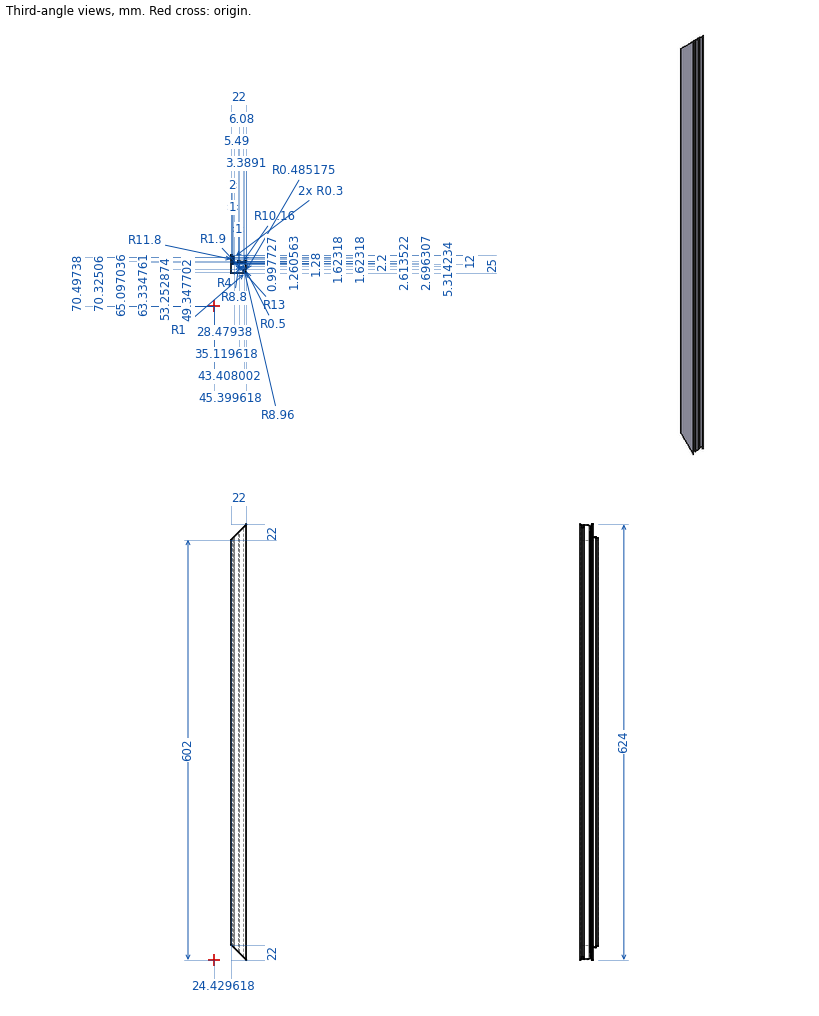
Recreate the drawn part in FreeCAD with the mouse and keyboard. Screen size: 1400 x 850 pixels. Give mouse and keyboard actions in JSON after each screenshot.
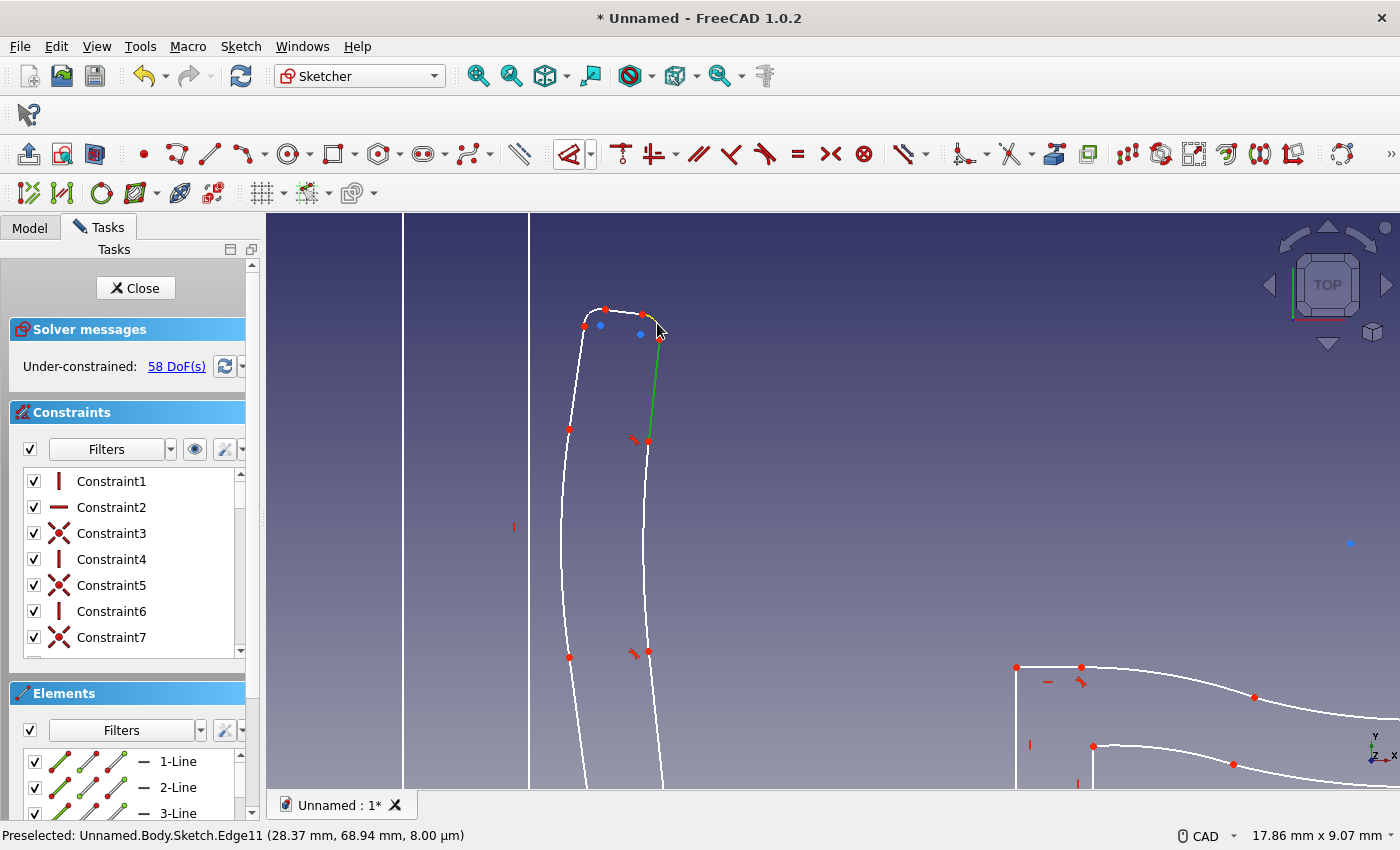
{"action": "left_click", "coordinate": [657, 323]}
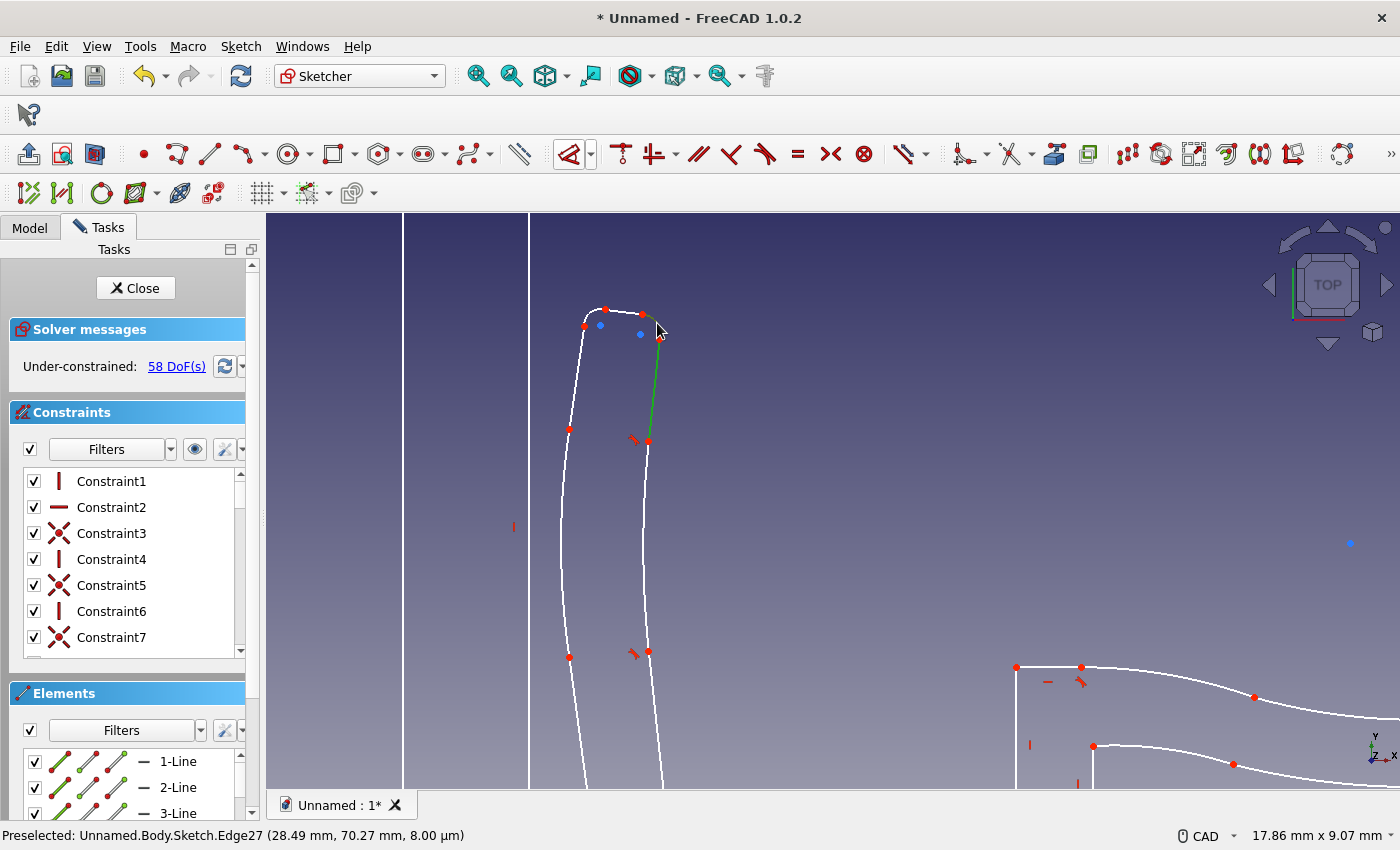
{"action": "key", "text": "t"}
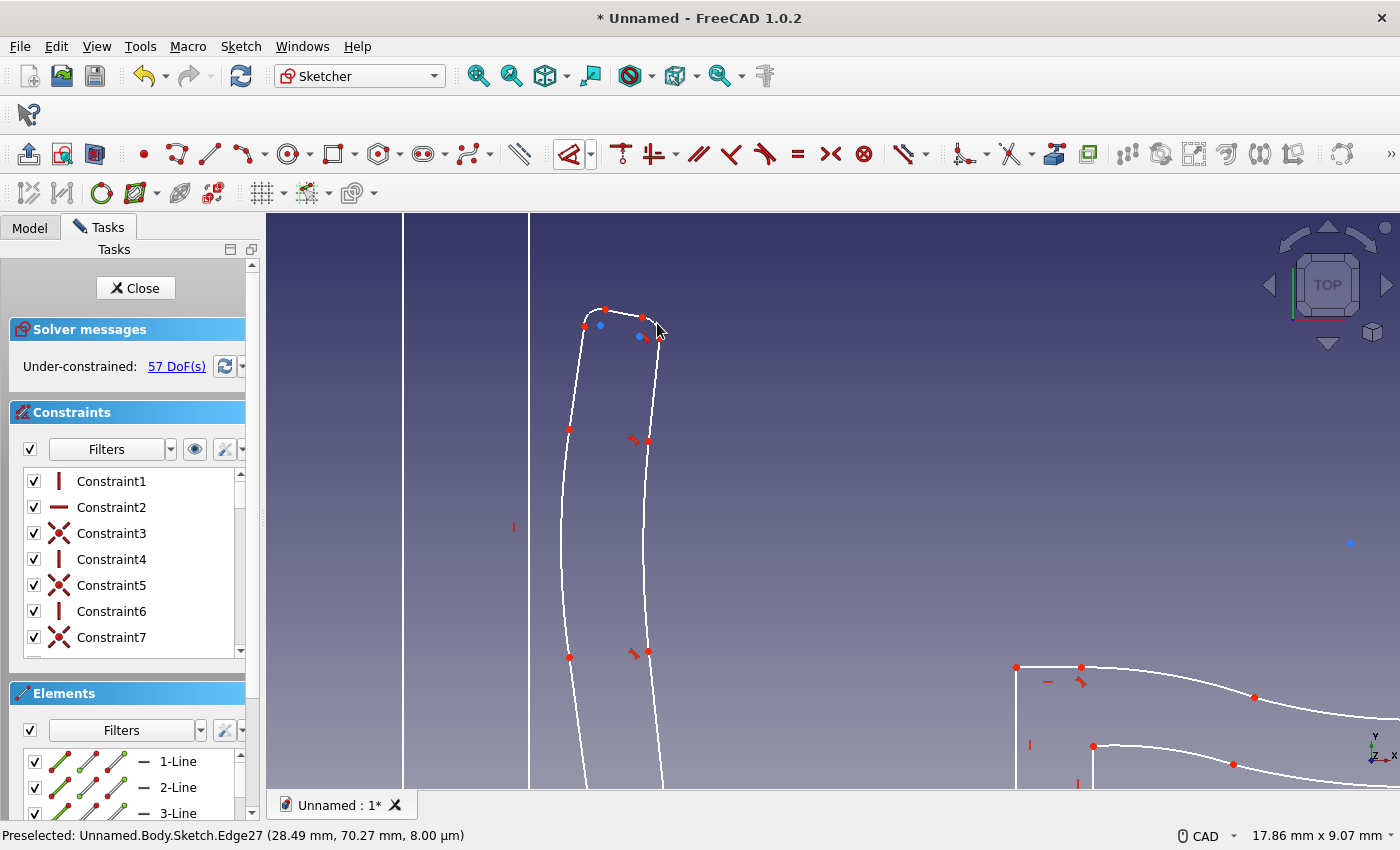
{"action": "left_click", "coordinate": [631, 315]}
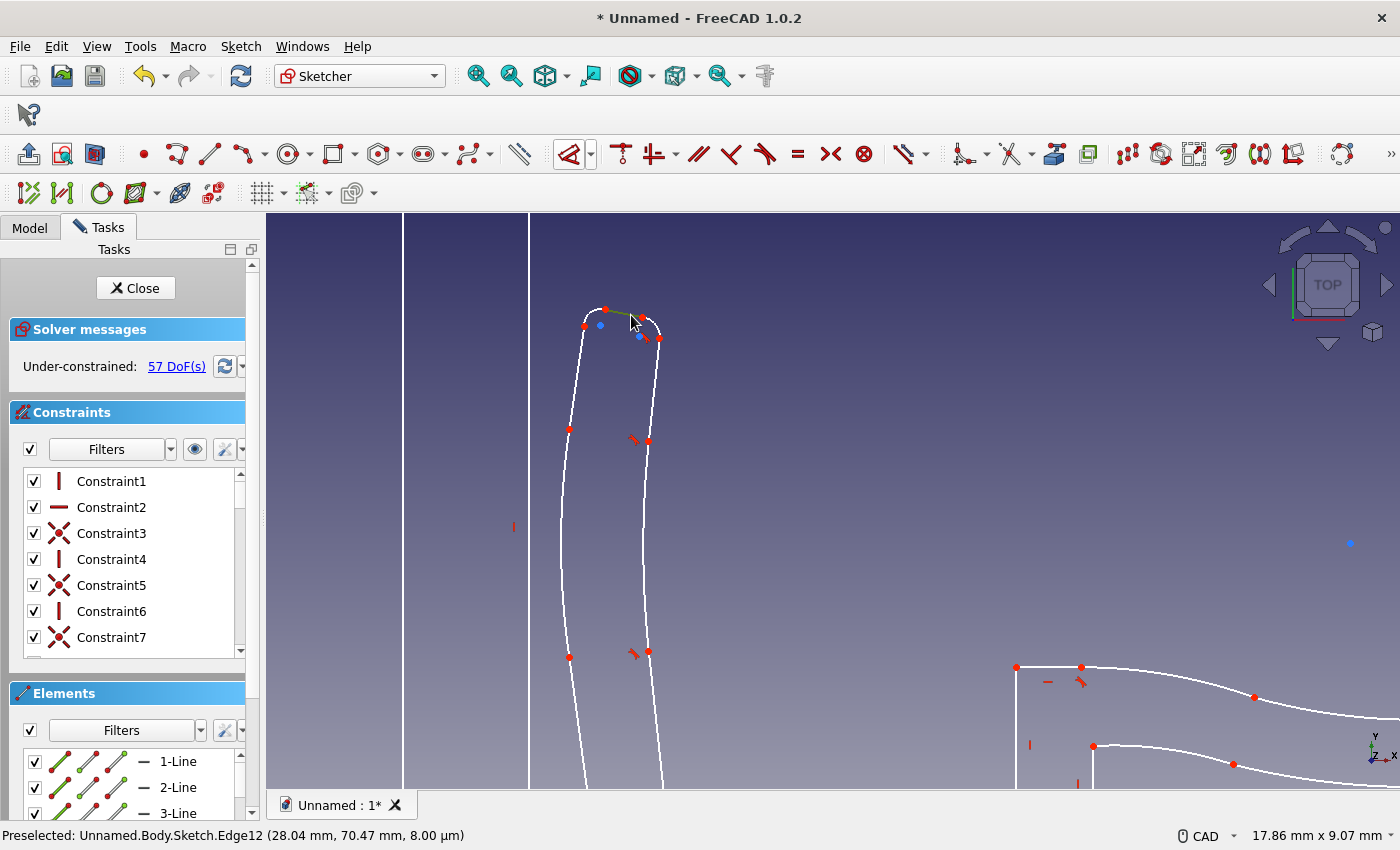
{"action": "scroll", "coordinate": [659, 330], "scroll_direction": "up", "scroll_amount": 3}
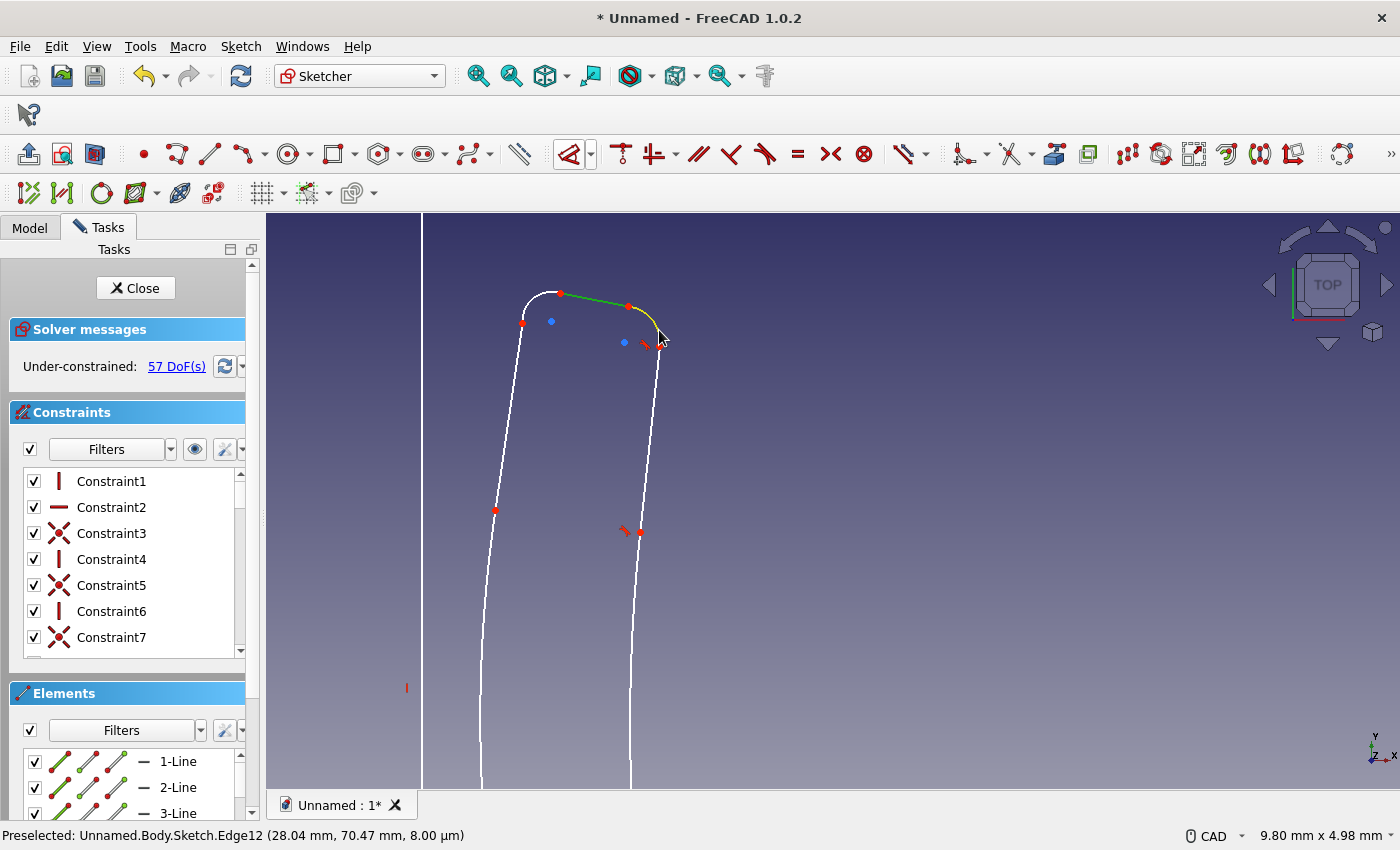
{"action": "left_click", "coordinate": [658, 330]}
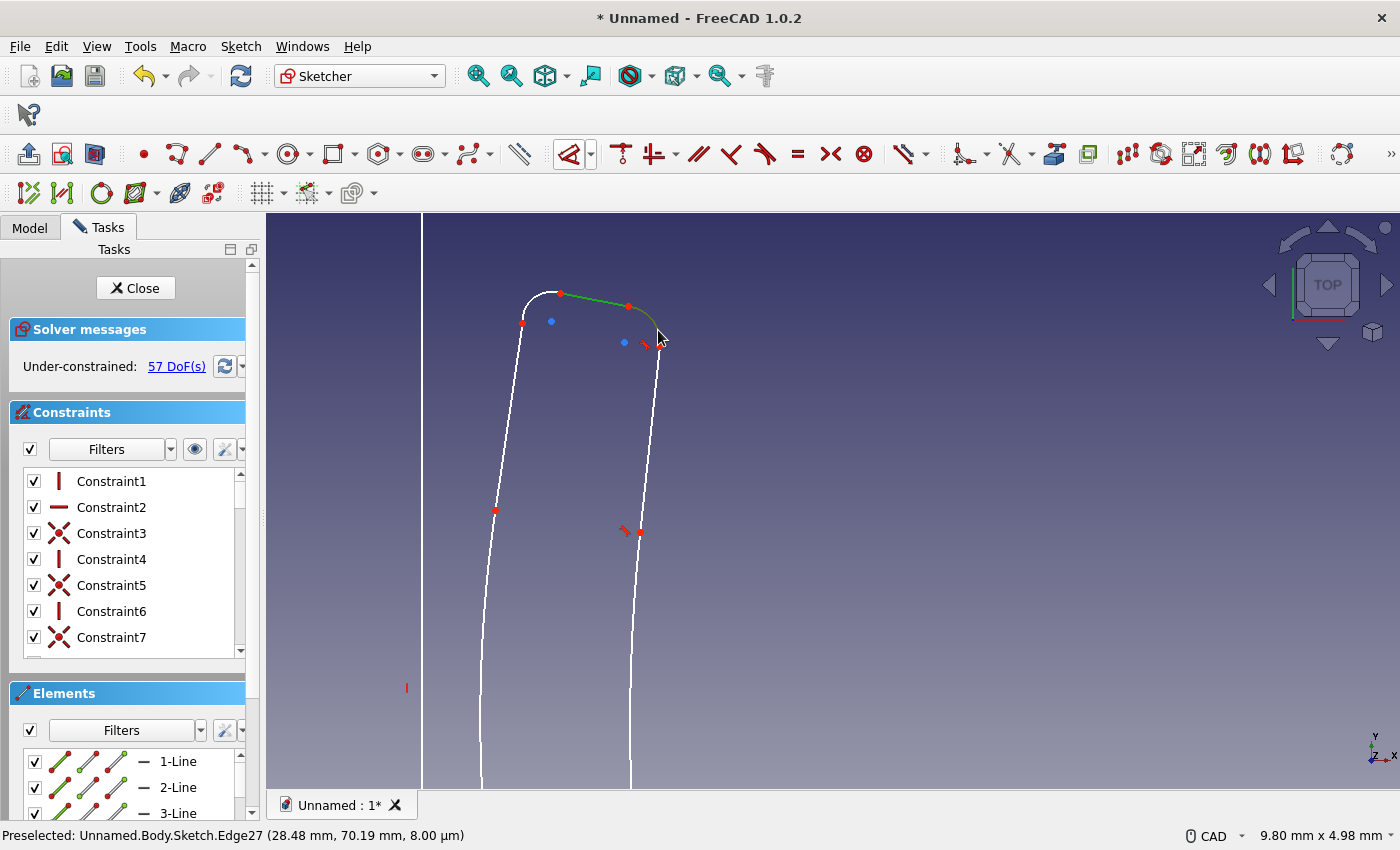
{"action": "key", "text": "t"}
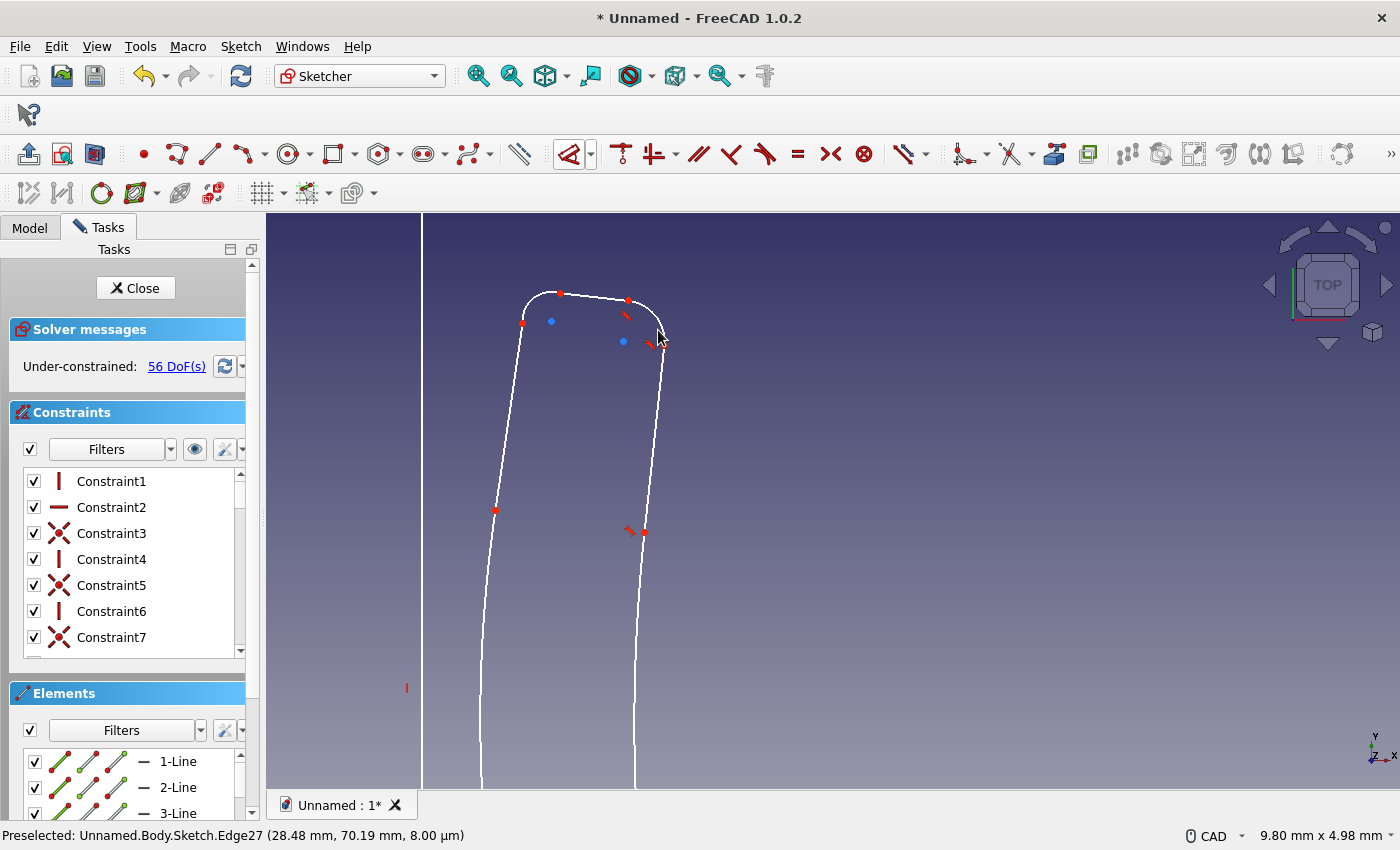
{"action": "left_click", "coordinate": [608, 299]}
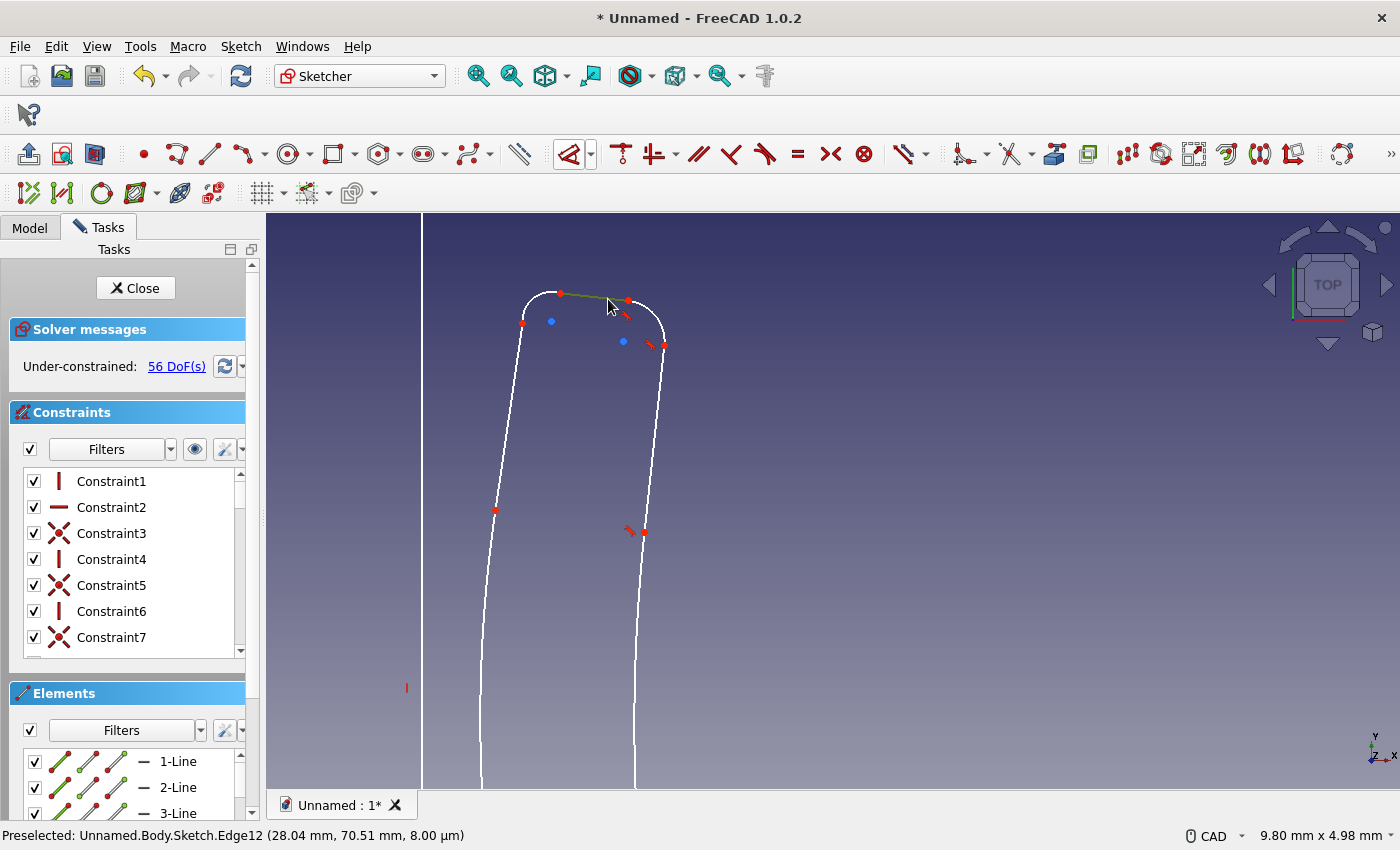
{"action": "left_click", "coordinate": [544, 293]}